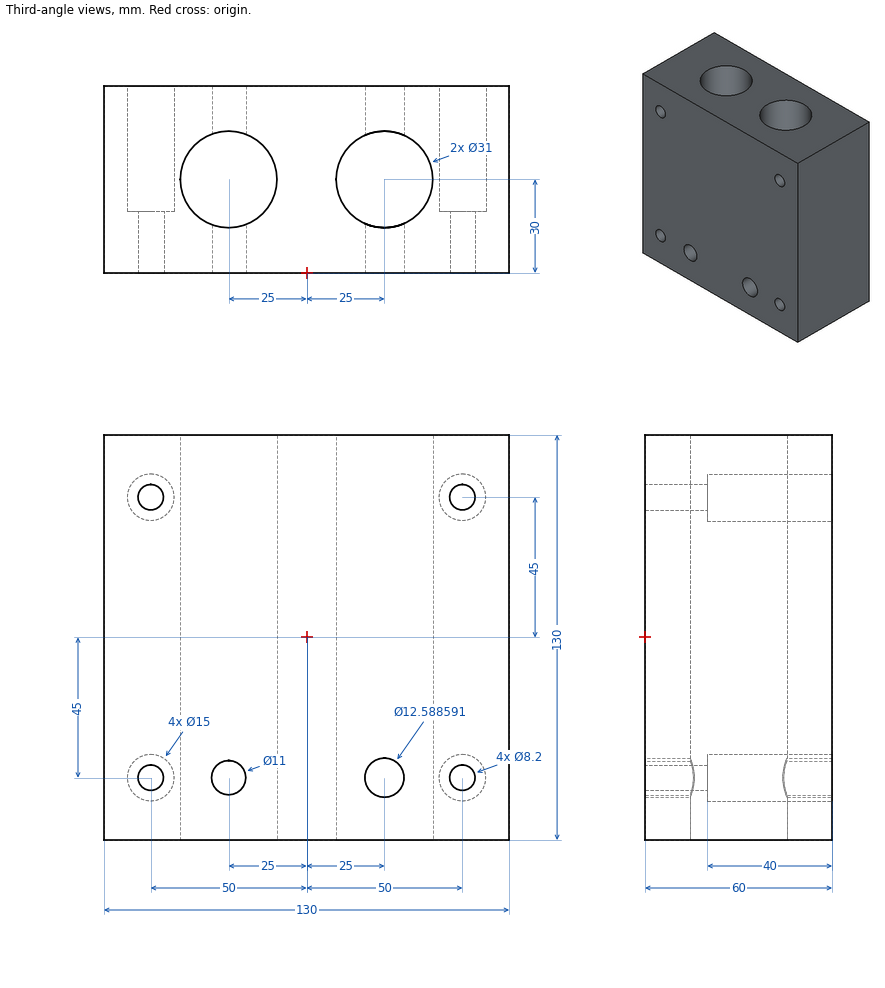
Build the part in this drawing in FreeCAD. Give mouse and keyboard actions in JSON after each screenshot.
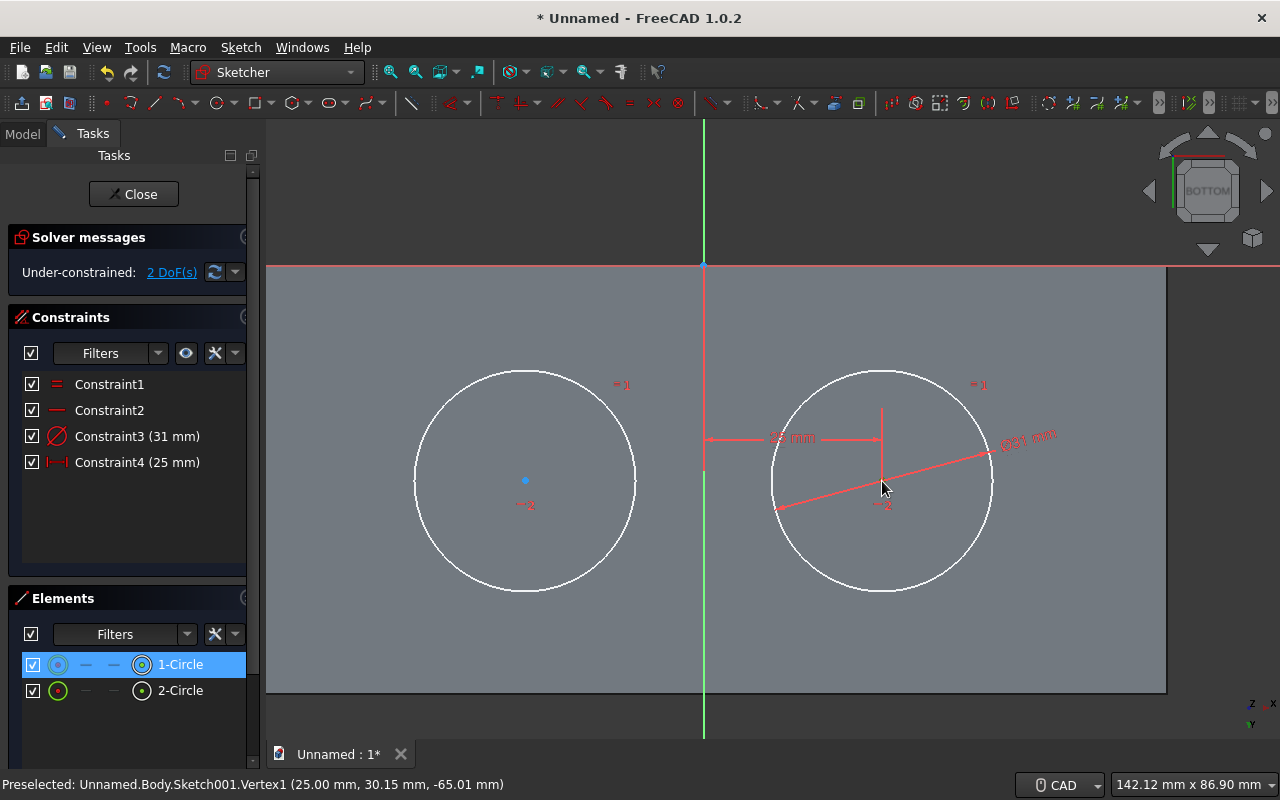
{"action": "key", "text": "i"}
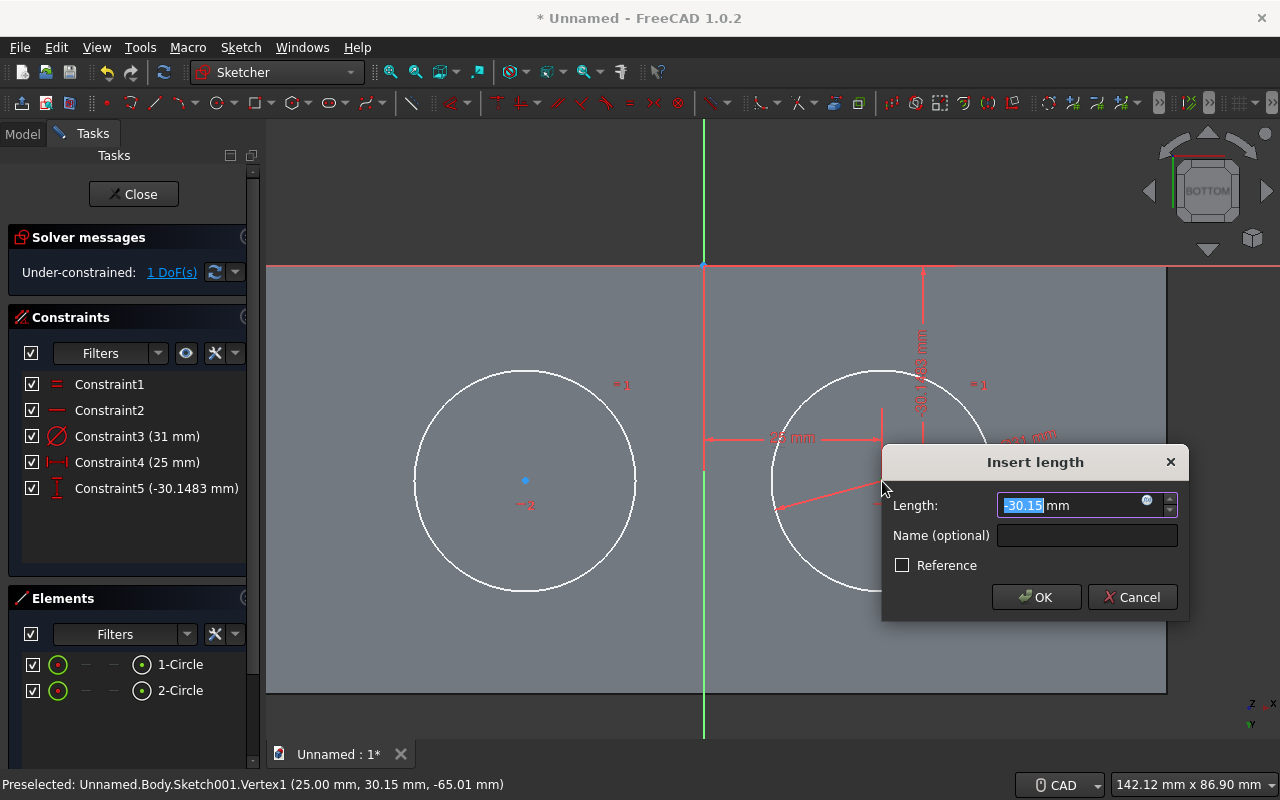
{"action": "type", "text": "-30"}
{"action": "key", "text": "Return"}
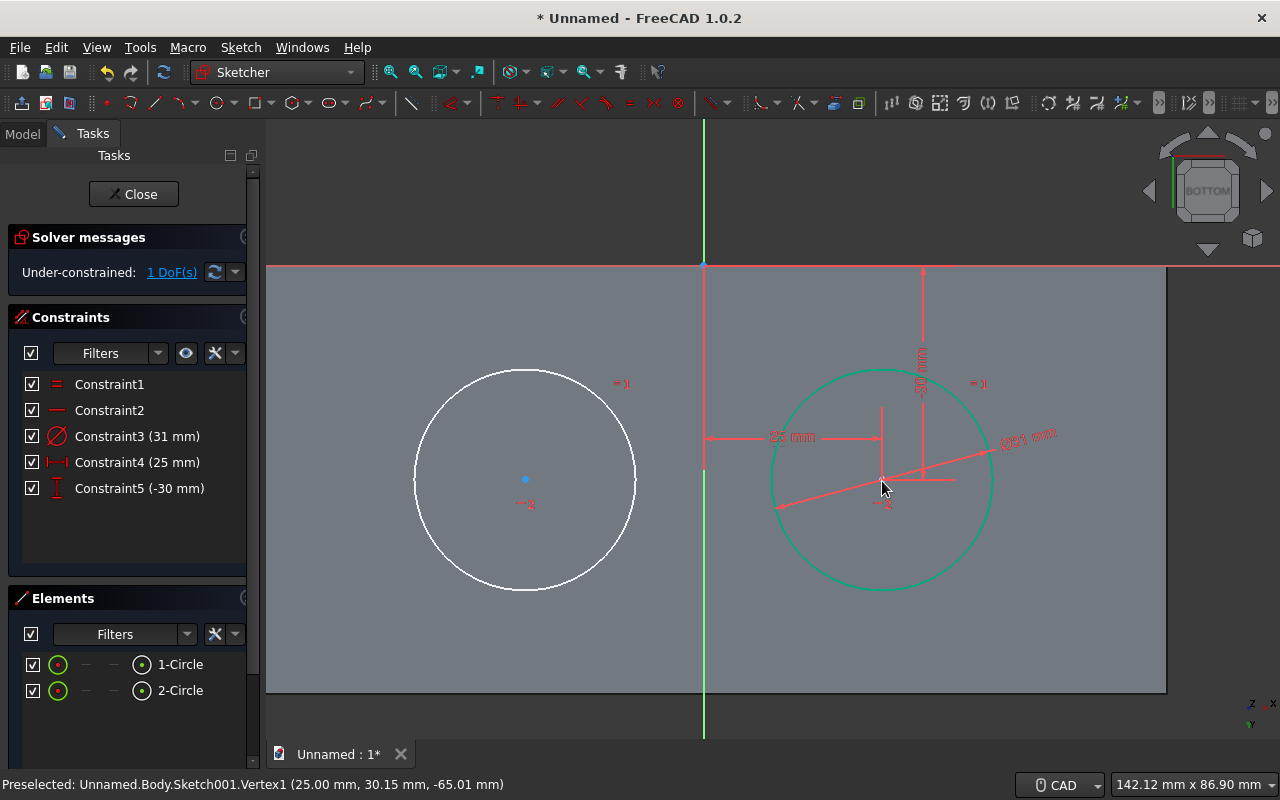
{"action": "left_click", "coordinate": [525, 480]}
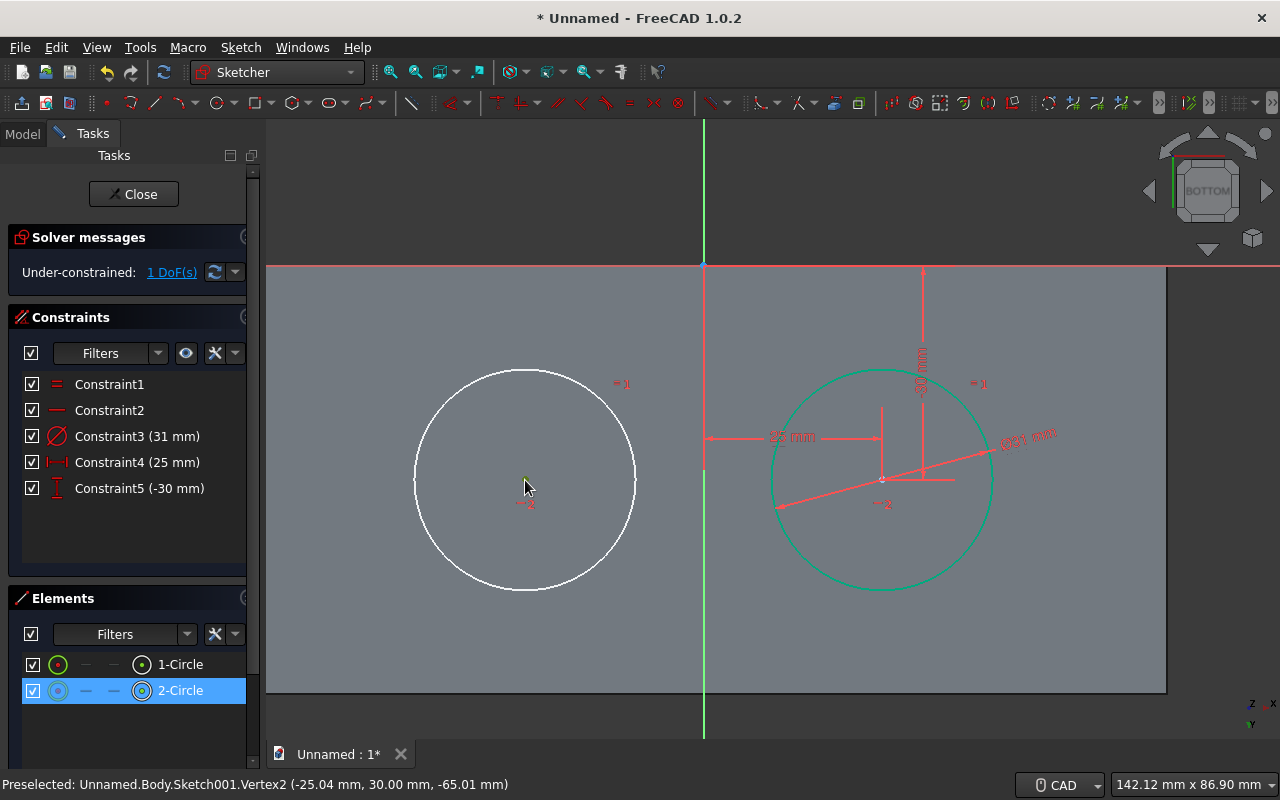
{"action": "key", "text": "l"}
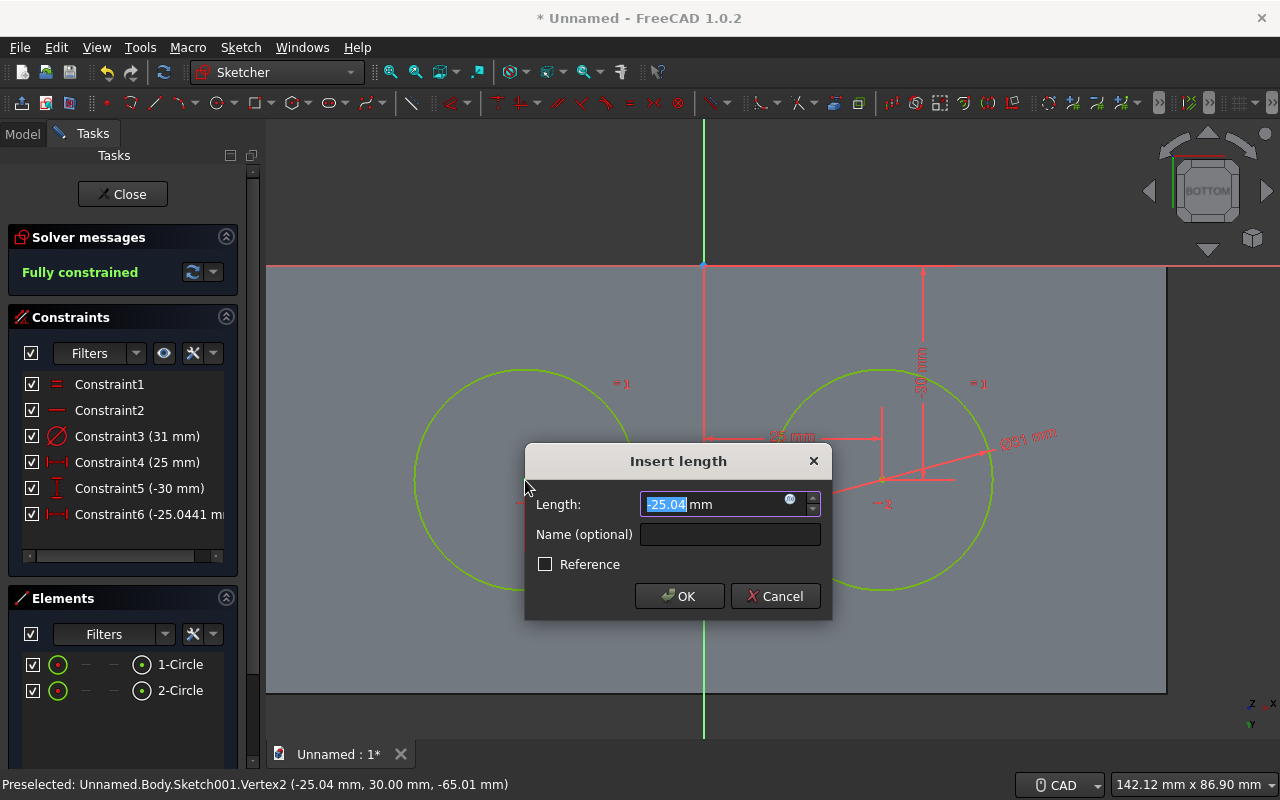
{"action": "type", "text": "-25"}
{"action": "key", "text": "Return"}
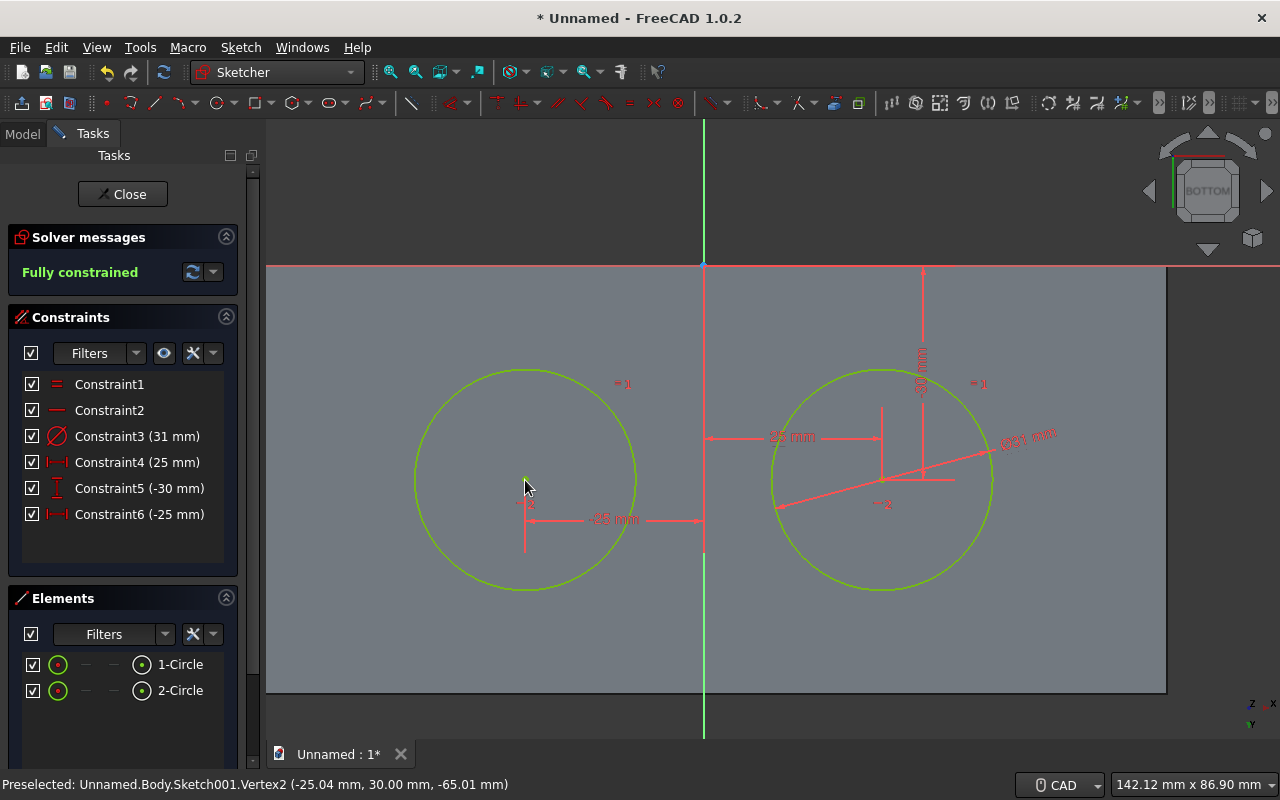
{"action": "left_click", "coordinate": [123, 194]}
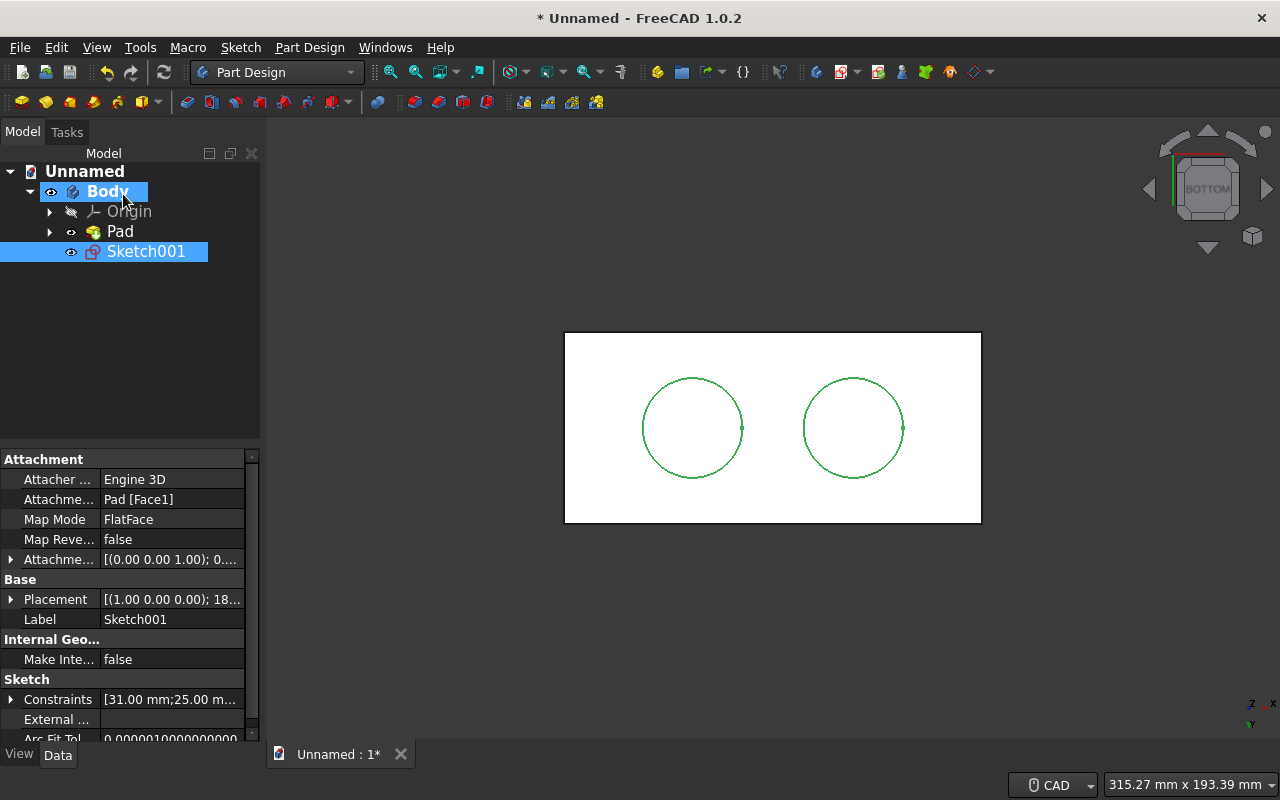
{"action": "left_click", "coordinate": [188, 102]}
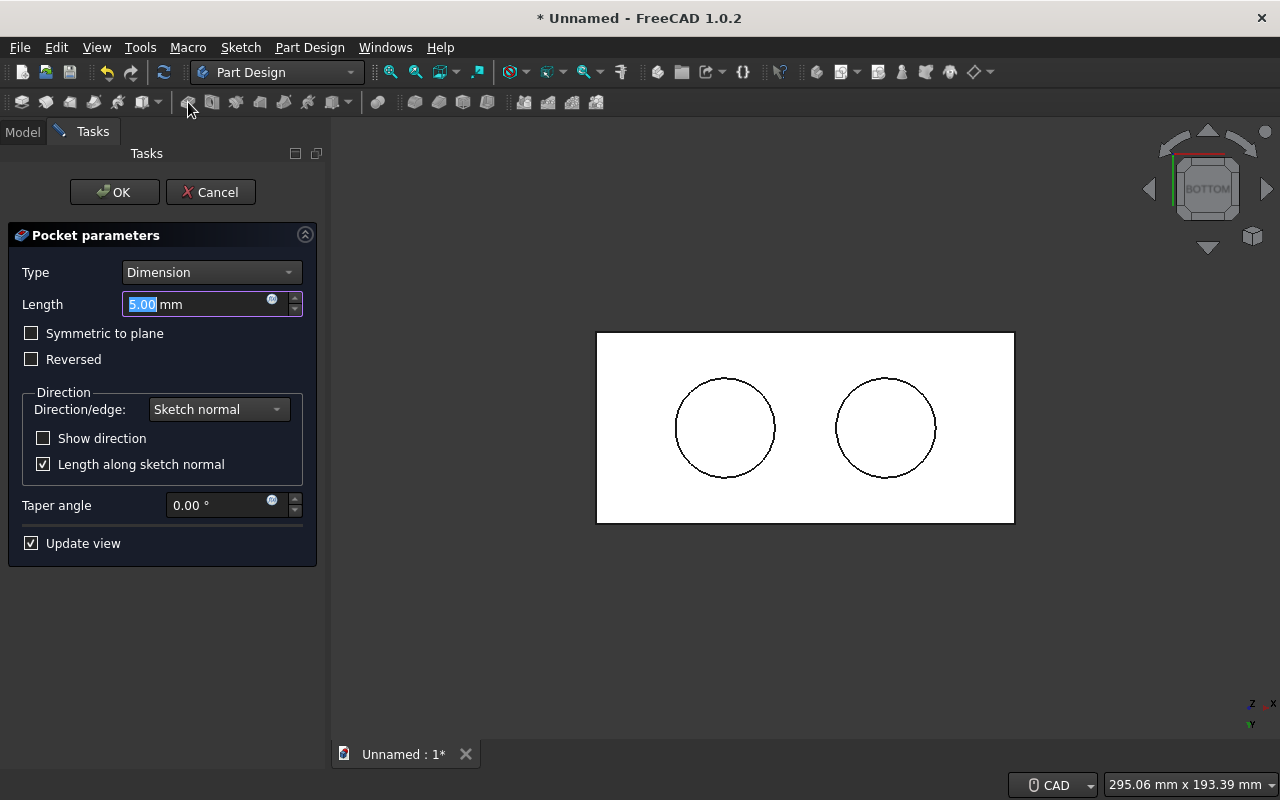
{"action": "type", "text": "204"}
{"action": "key", "text": "Tab"}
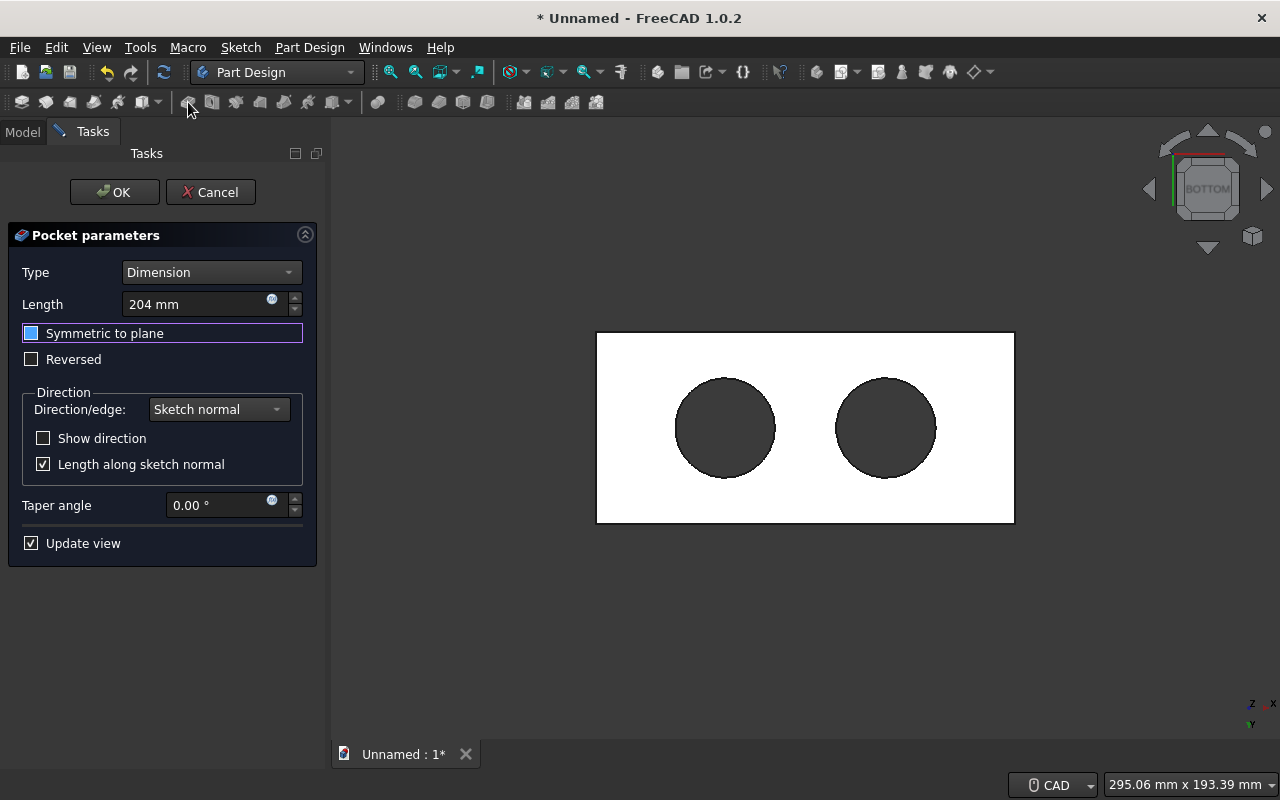
{"action": "left_click", "coordinate": [115, 192]}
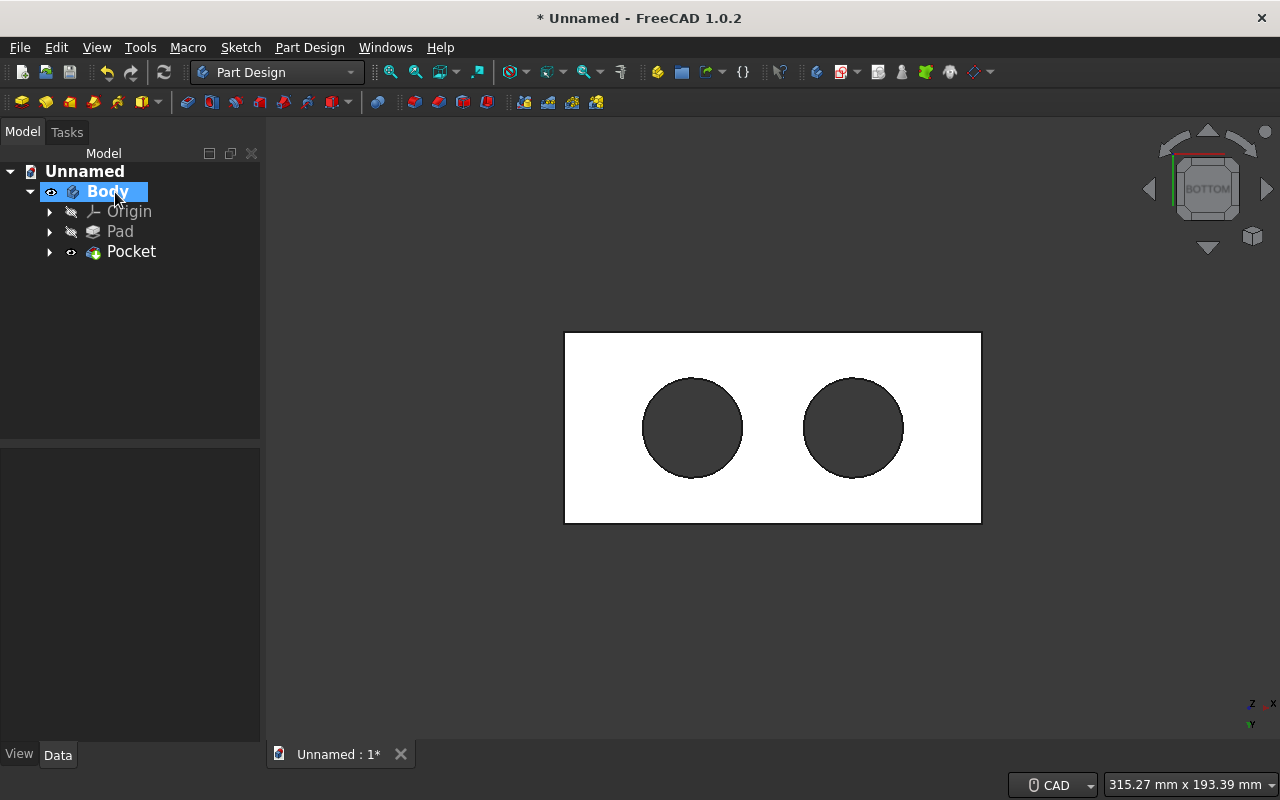
{"action": "key", "text": "v f"}